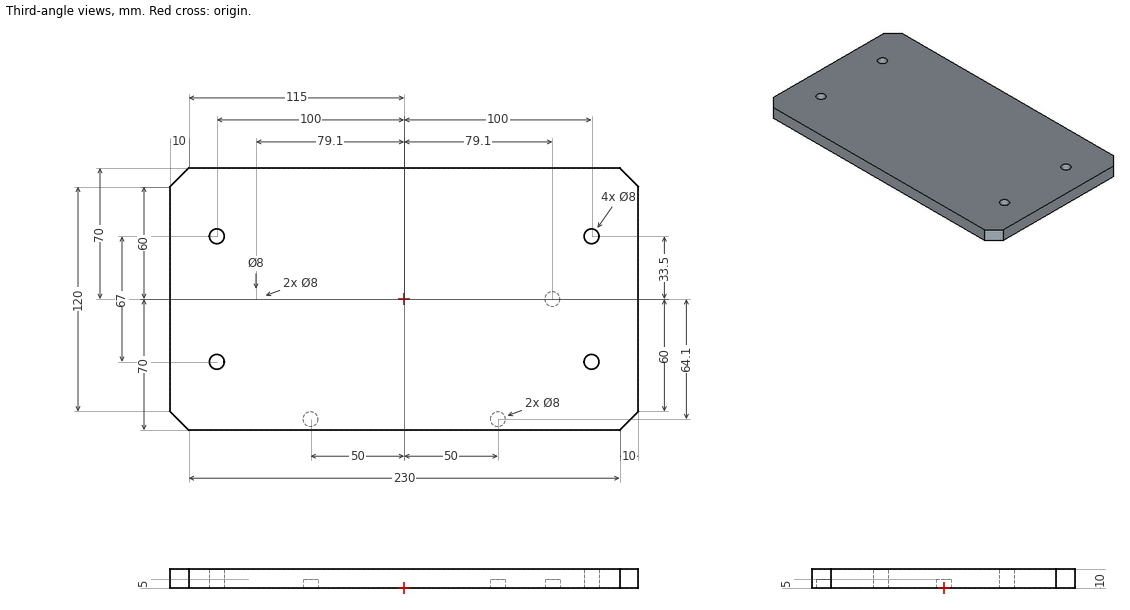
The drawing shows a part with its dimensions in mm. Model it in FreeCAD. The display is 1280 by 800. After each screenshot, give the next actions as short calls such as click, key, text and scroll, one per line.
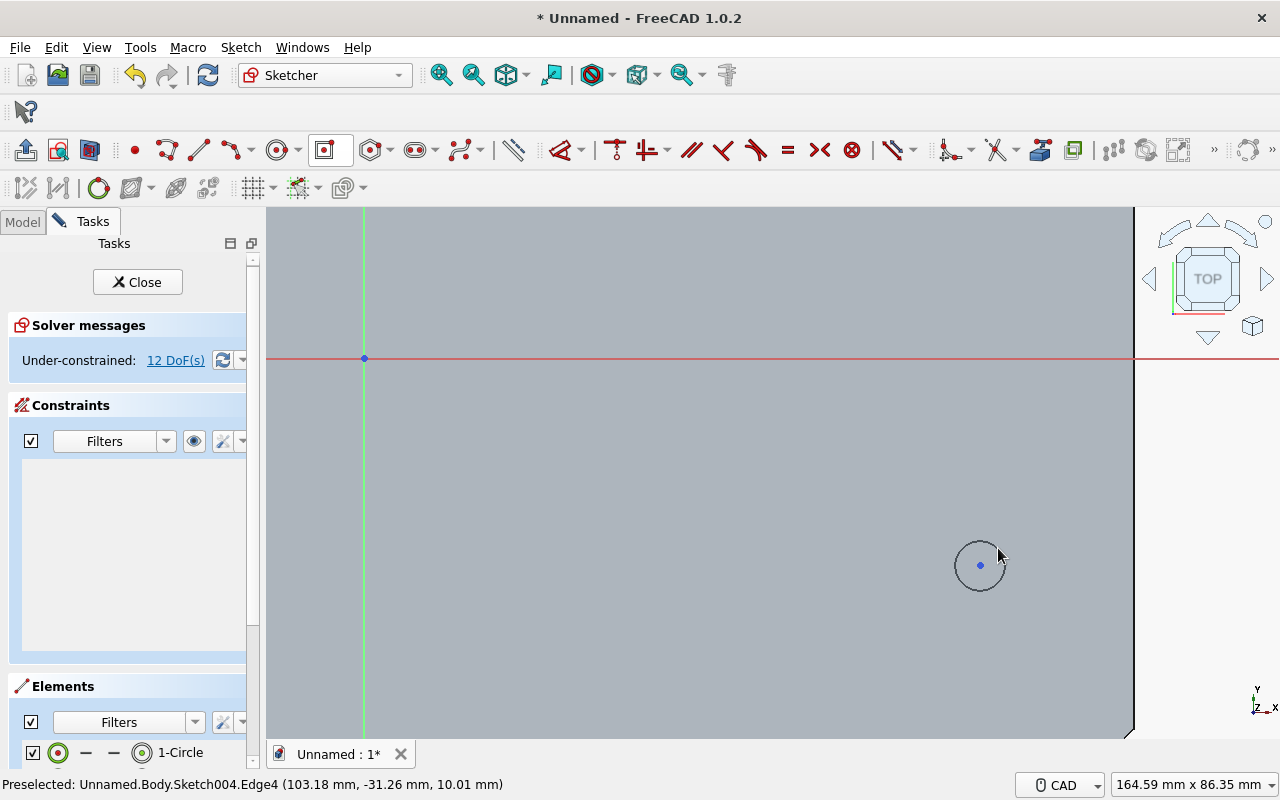
scroll(982, 566, down, 4)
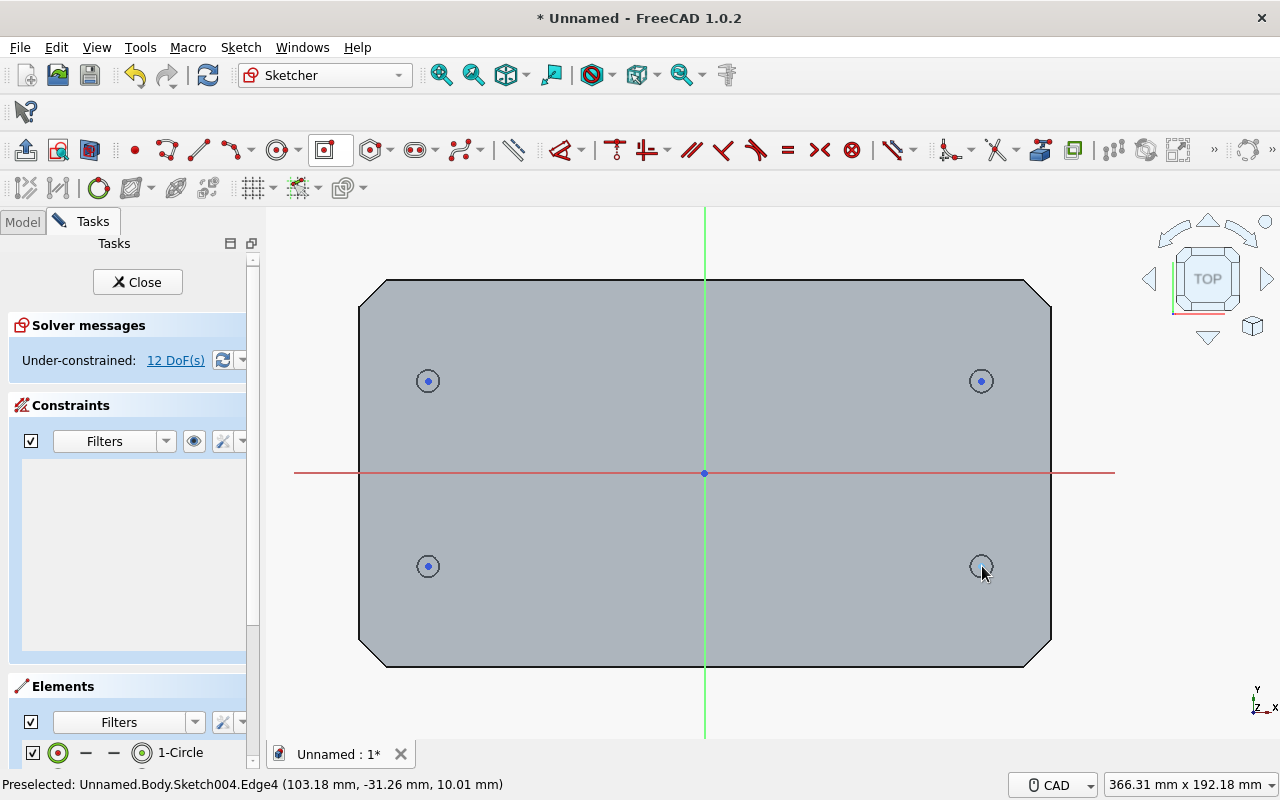
click(990, 373)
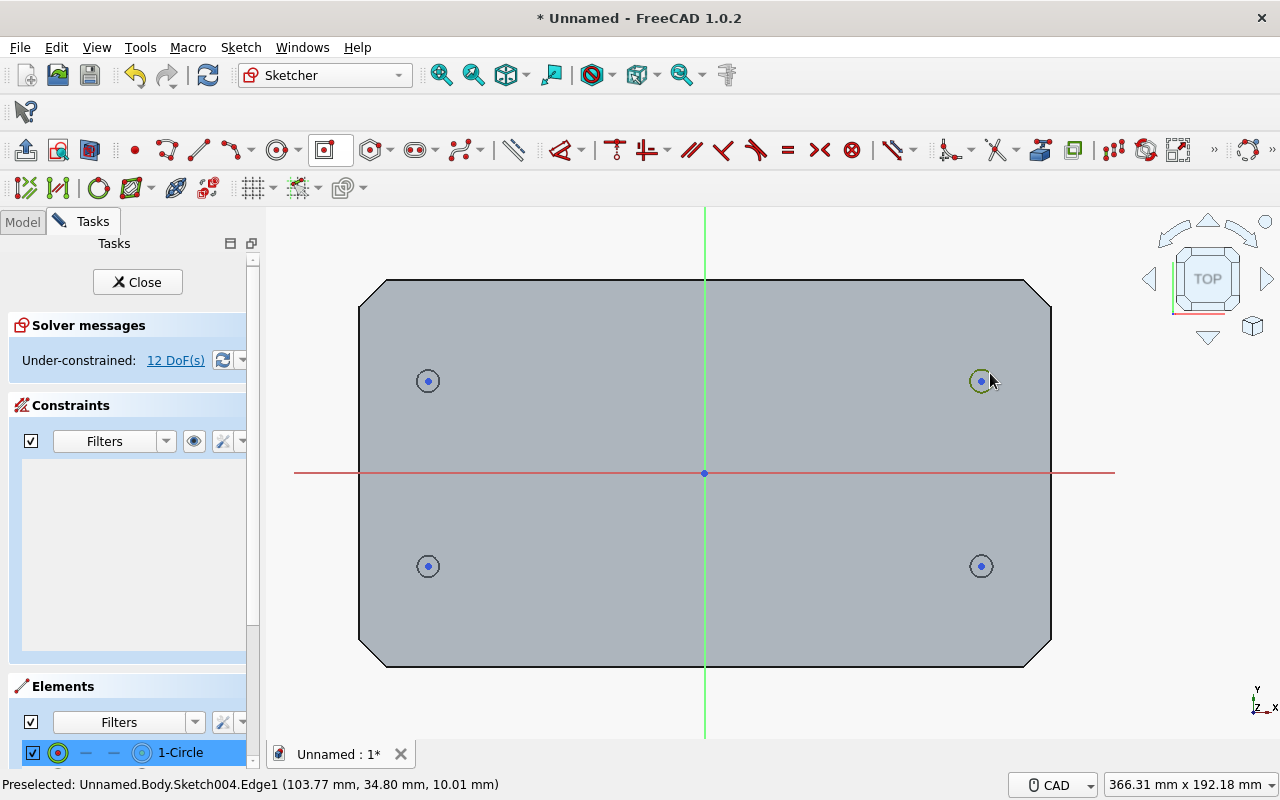
scroll(436, 373, up, 2)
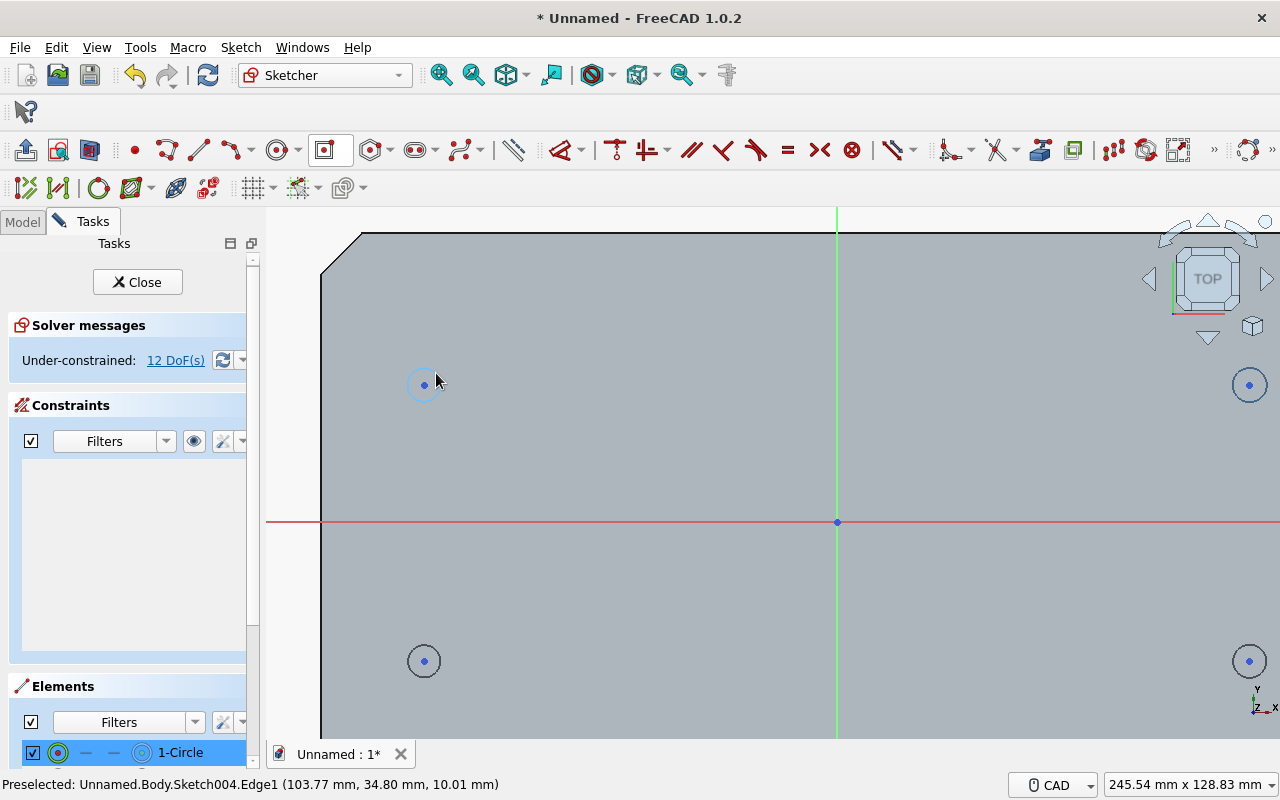
click(436, 373)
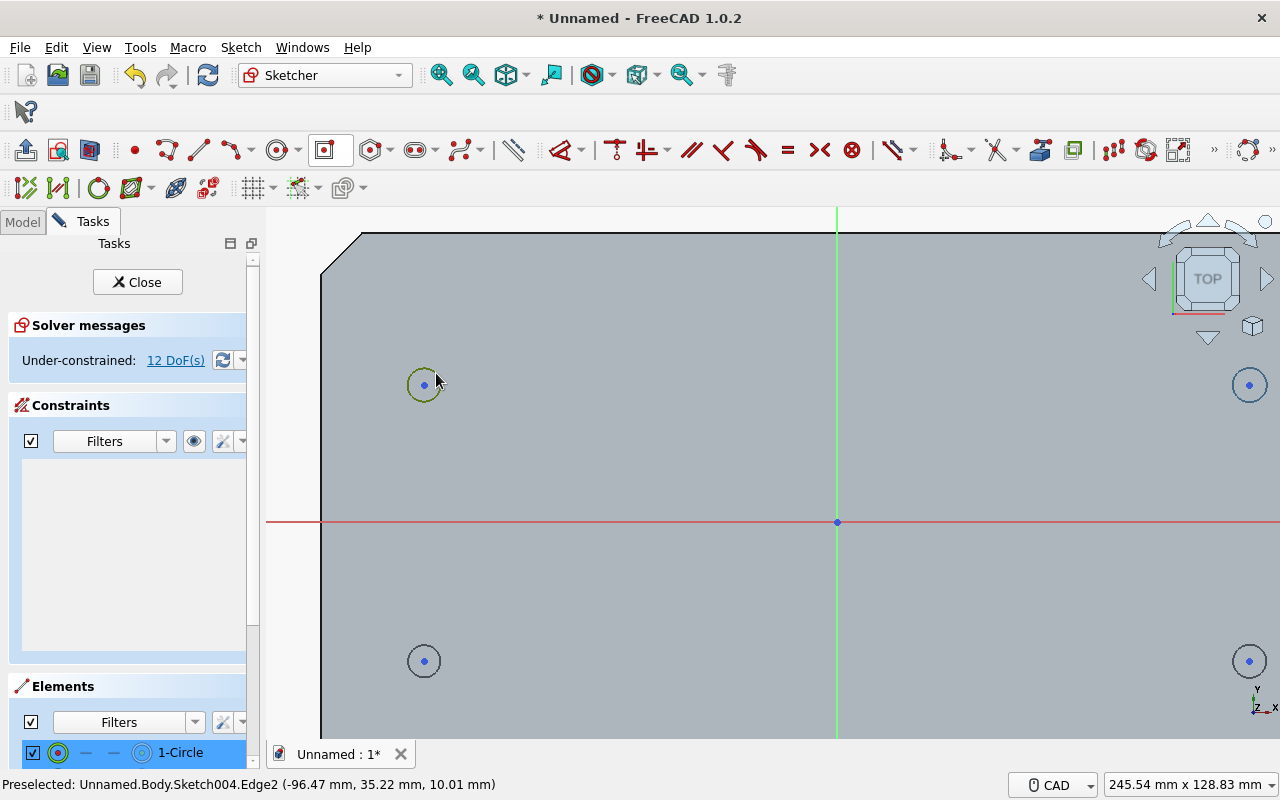
click(436, 650)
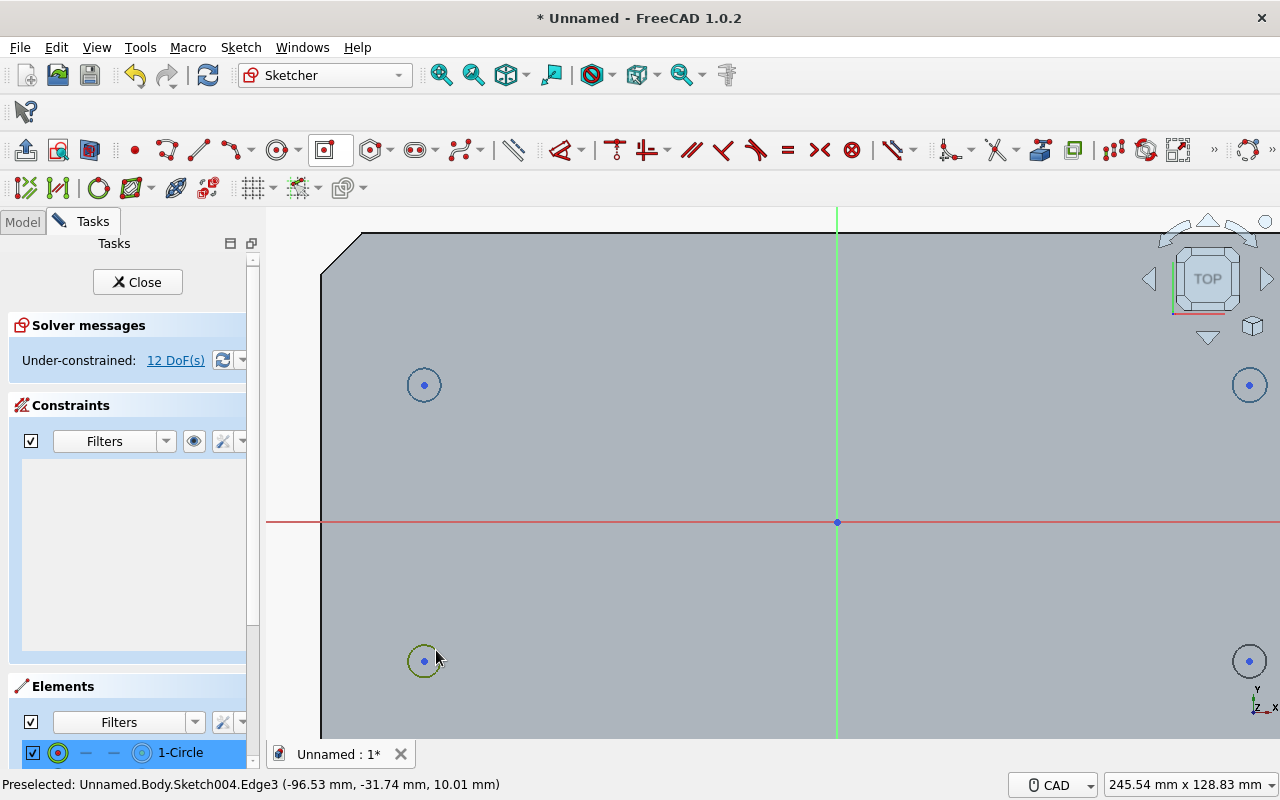
scroll(435, 372, down, 2)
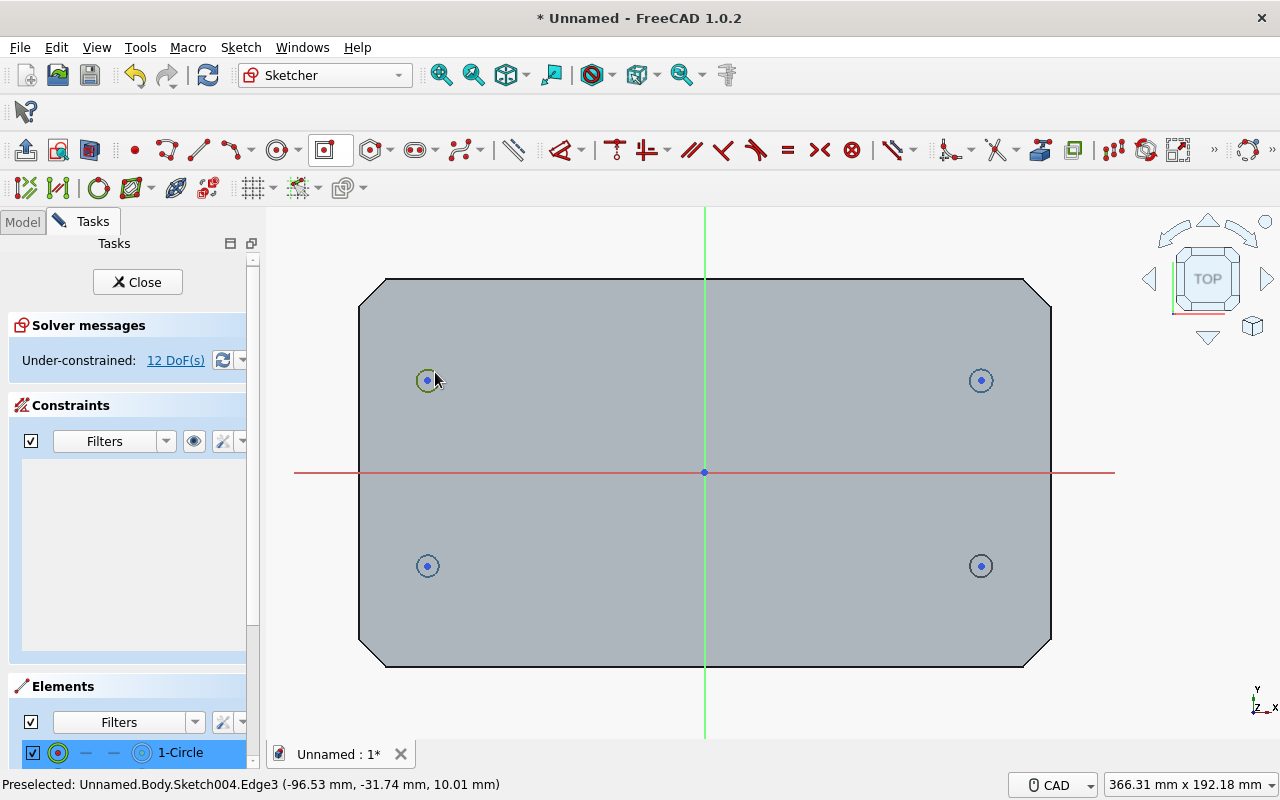
scroll(989, 558, up, 2)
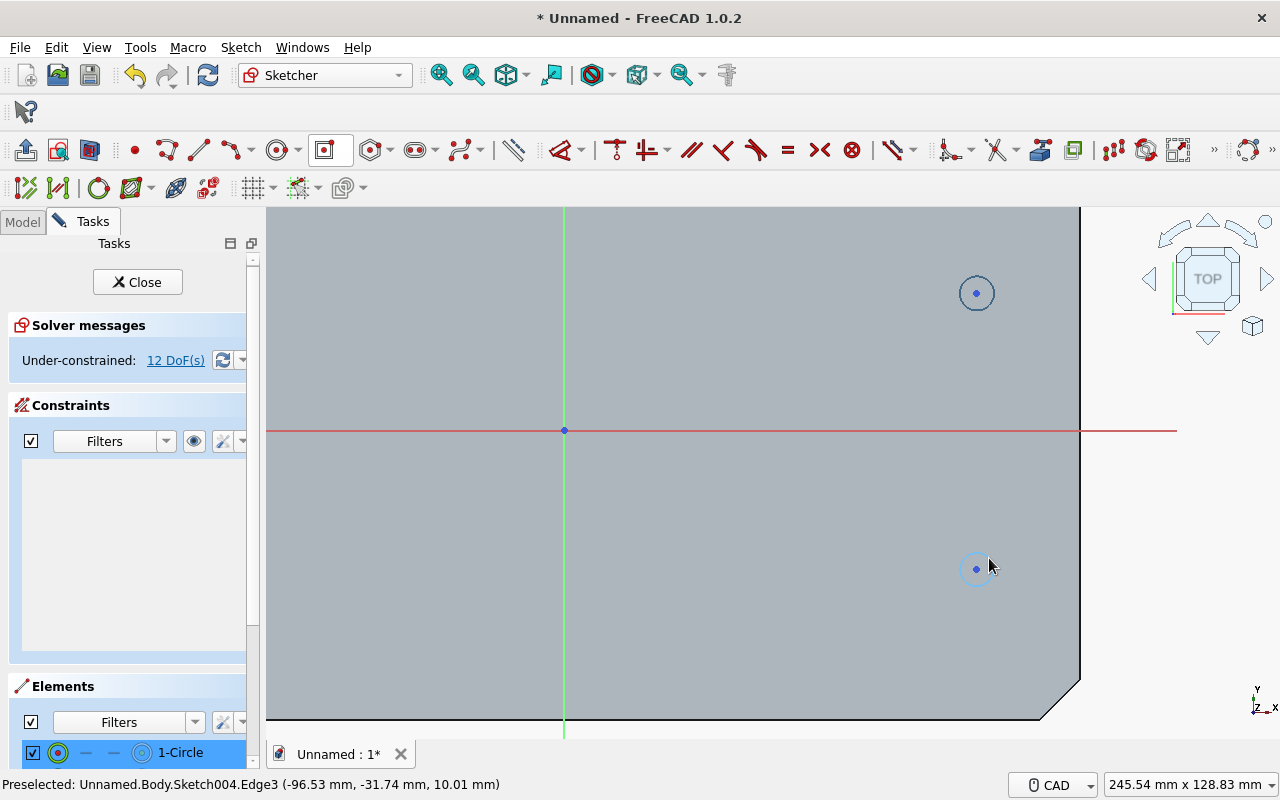
click(989, 558)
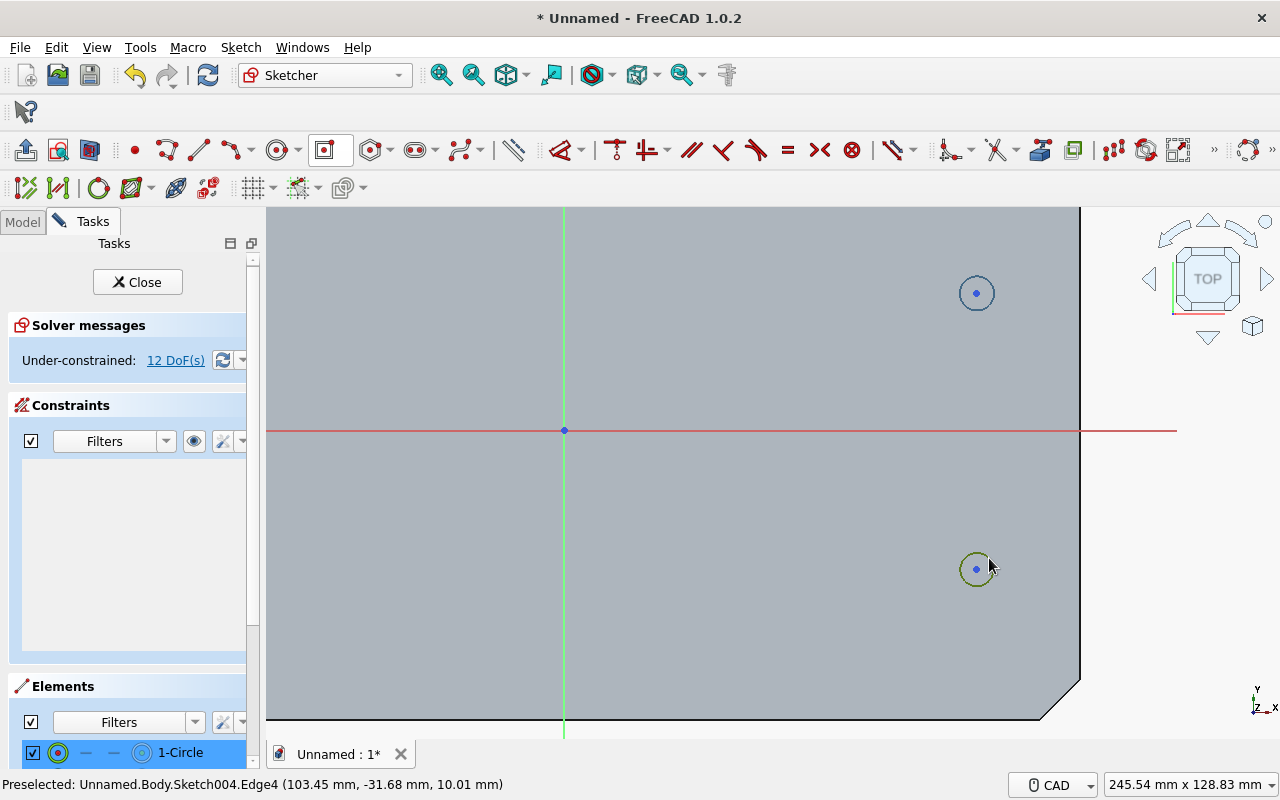
click(788, 150)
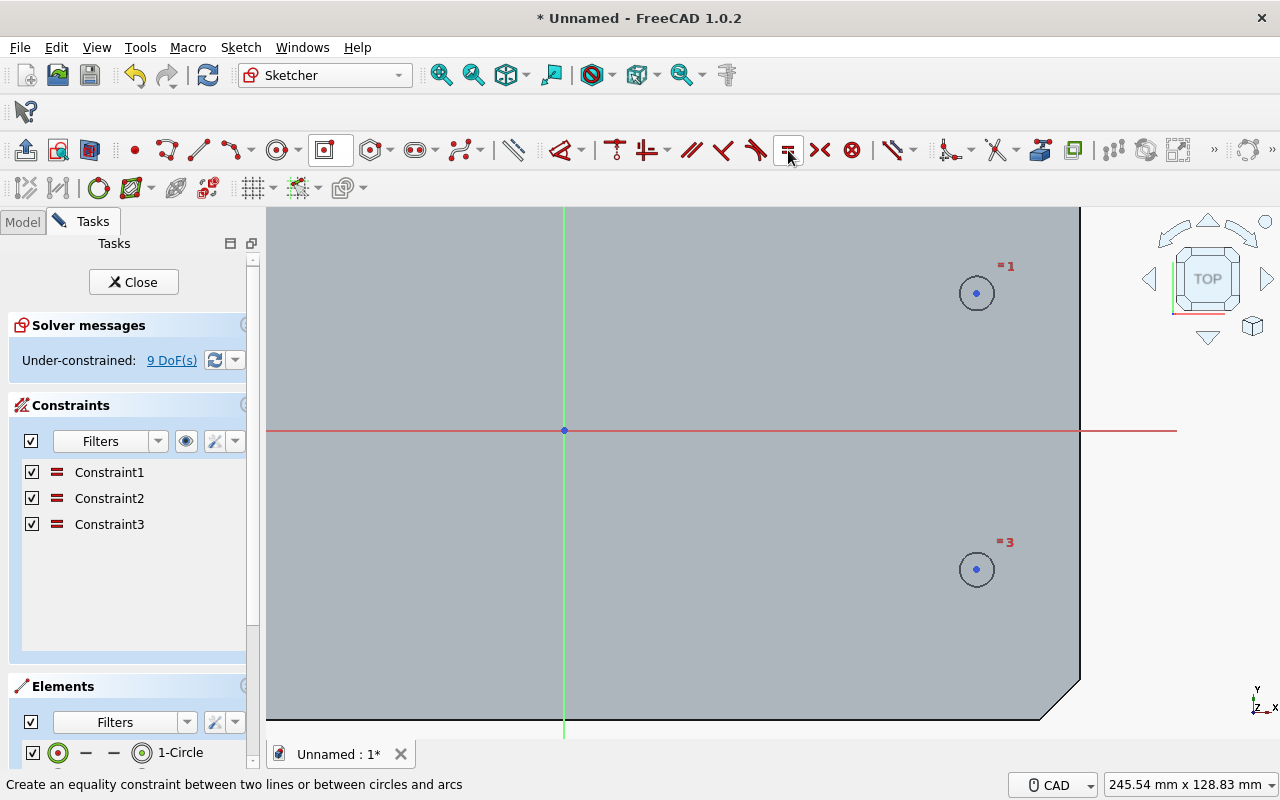
click(977, 293)